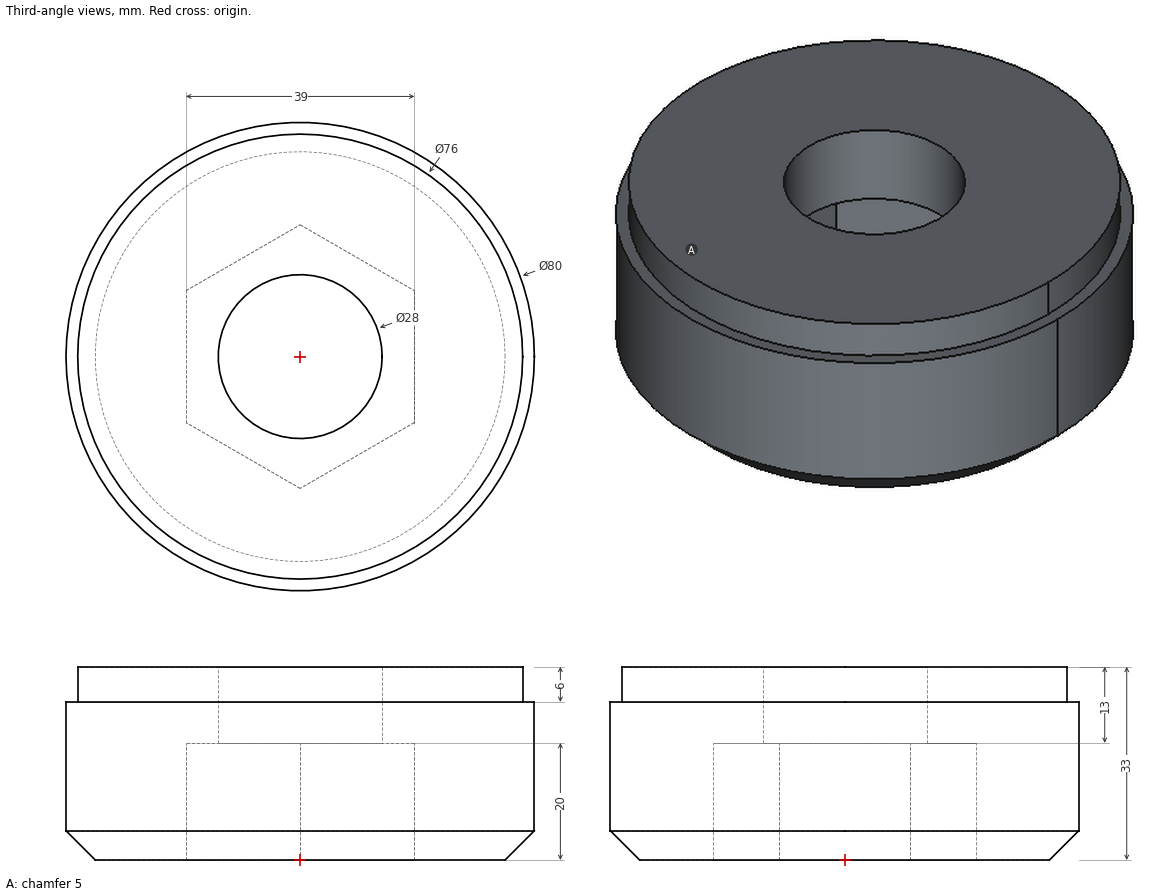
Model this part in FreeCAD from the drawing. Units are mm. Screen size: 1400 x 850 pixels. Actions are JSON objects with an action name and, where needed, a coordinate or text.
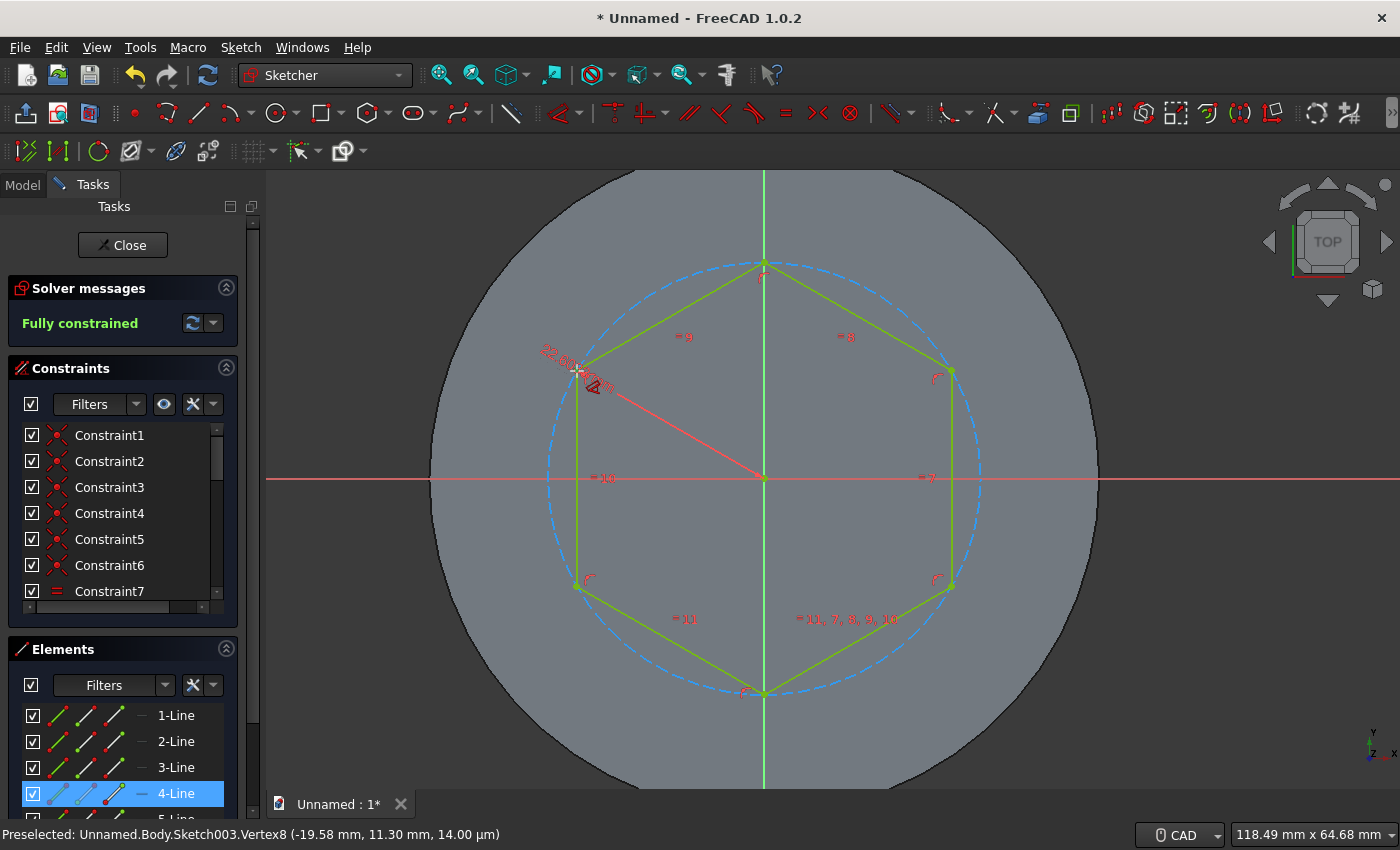
{"action": "left_click", "coordinate": [952, 587]}
{"action": "left_click", "coordinate": [678, 337]}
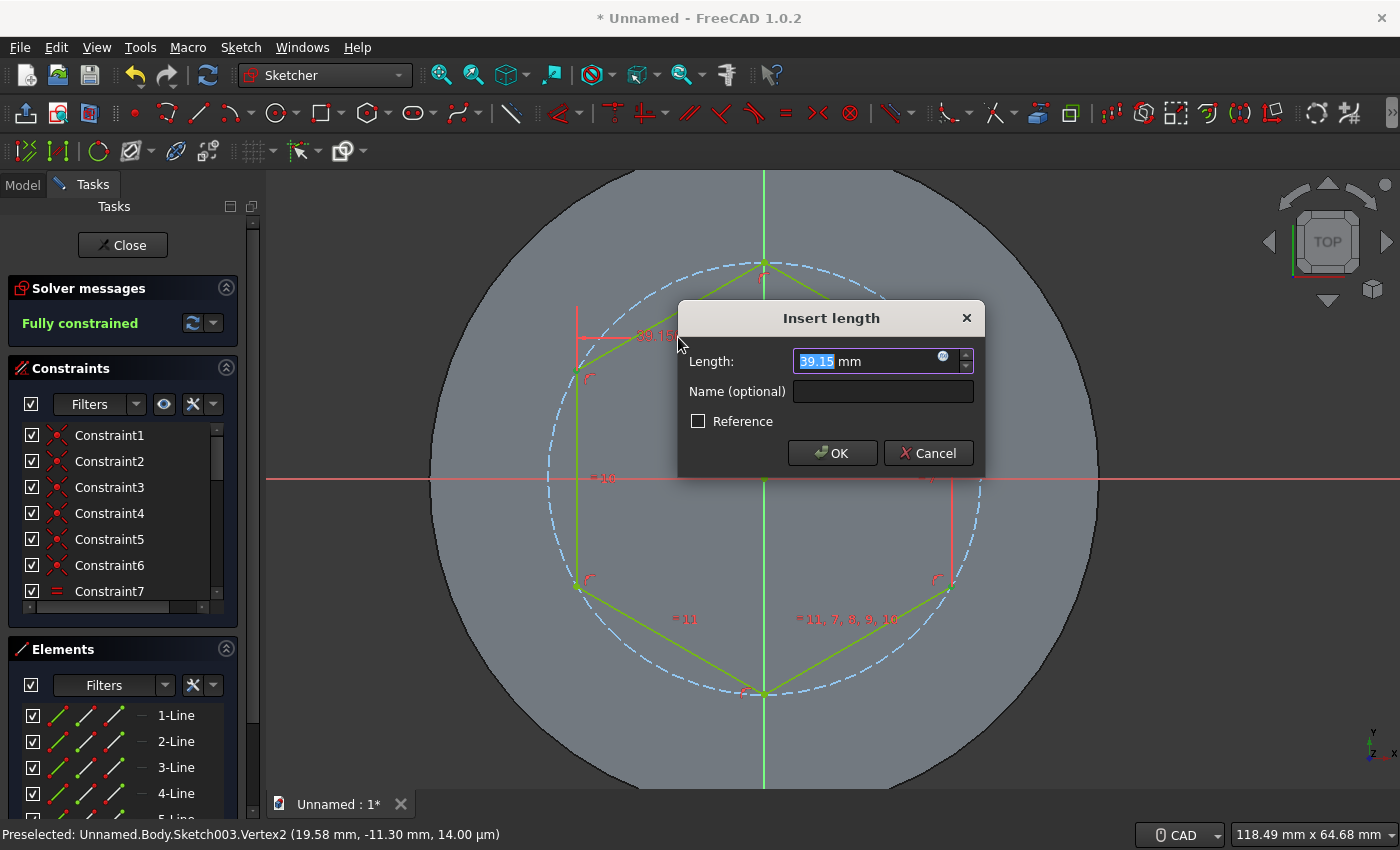
{"action": "type", "text": "39"}
{"action": "key", "text": "Return"}
{"action": "key", "text": "Escape"}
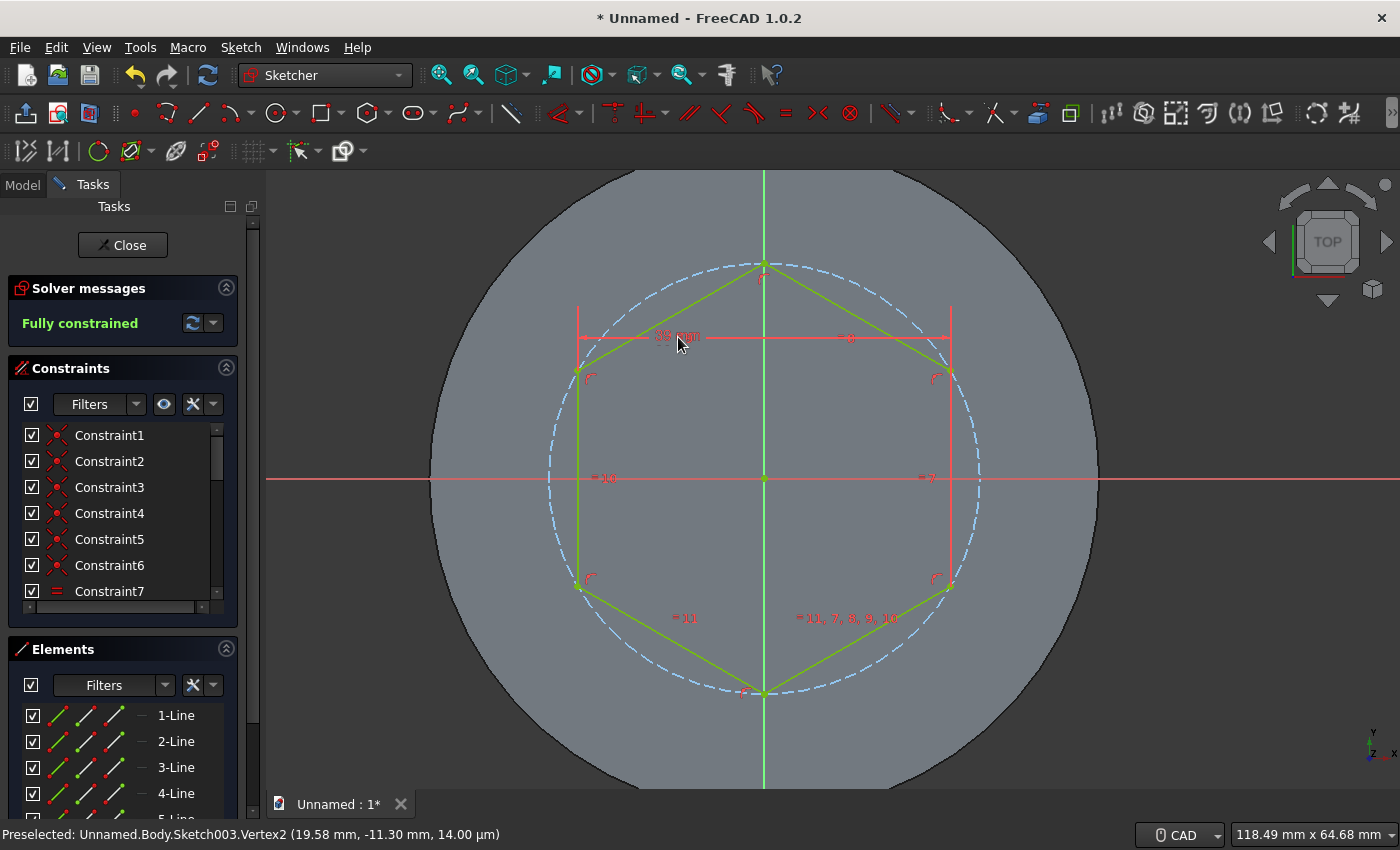
{"action": "left_click", "coordinate": [123, 245]}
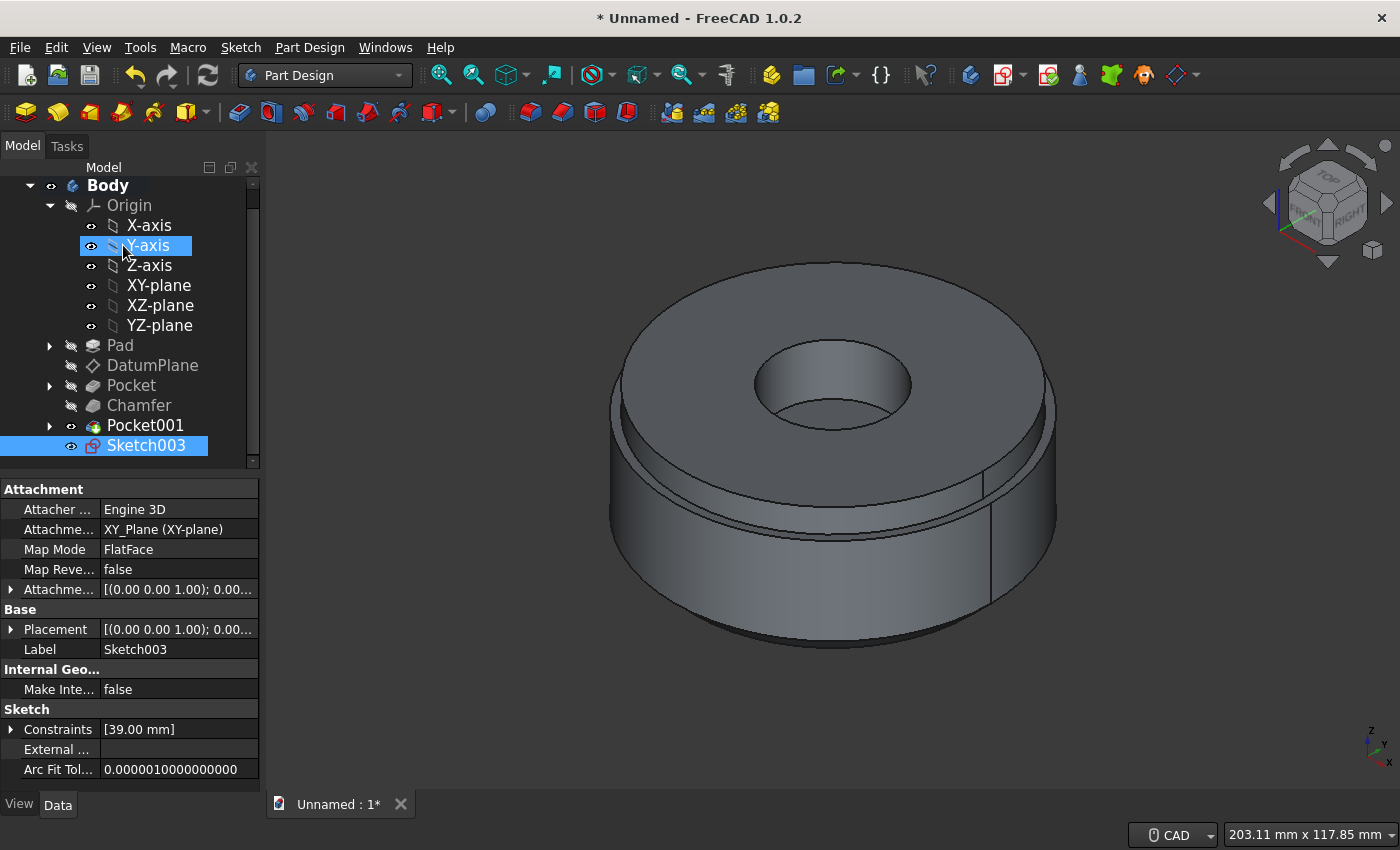
{"action": "left_click", "coordinate": [240, 112]}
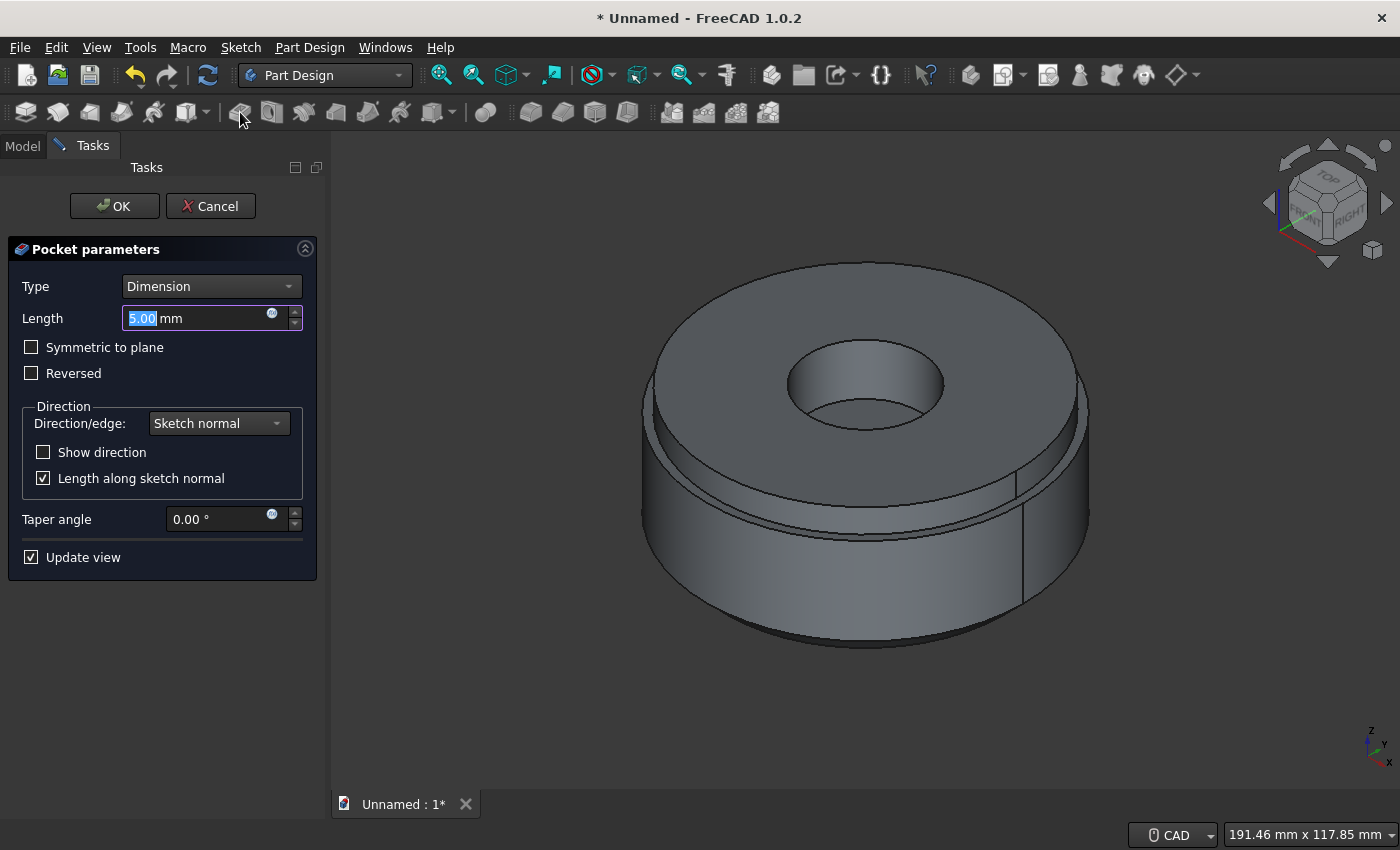
{"action": "type", "text": "20"}
{"action": "key", "text": "Tab"}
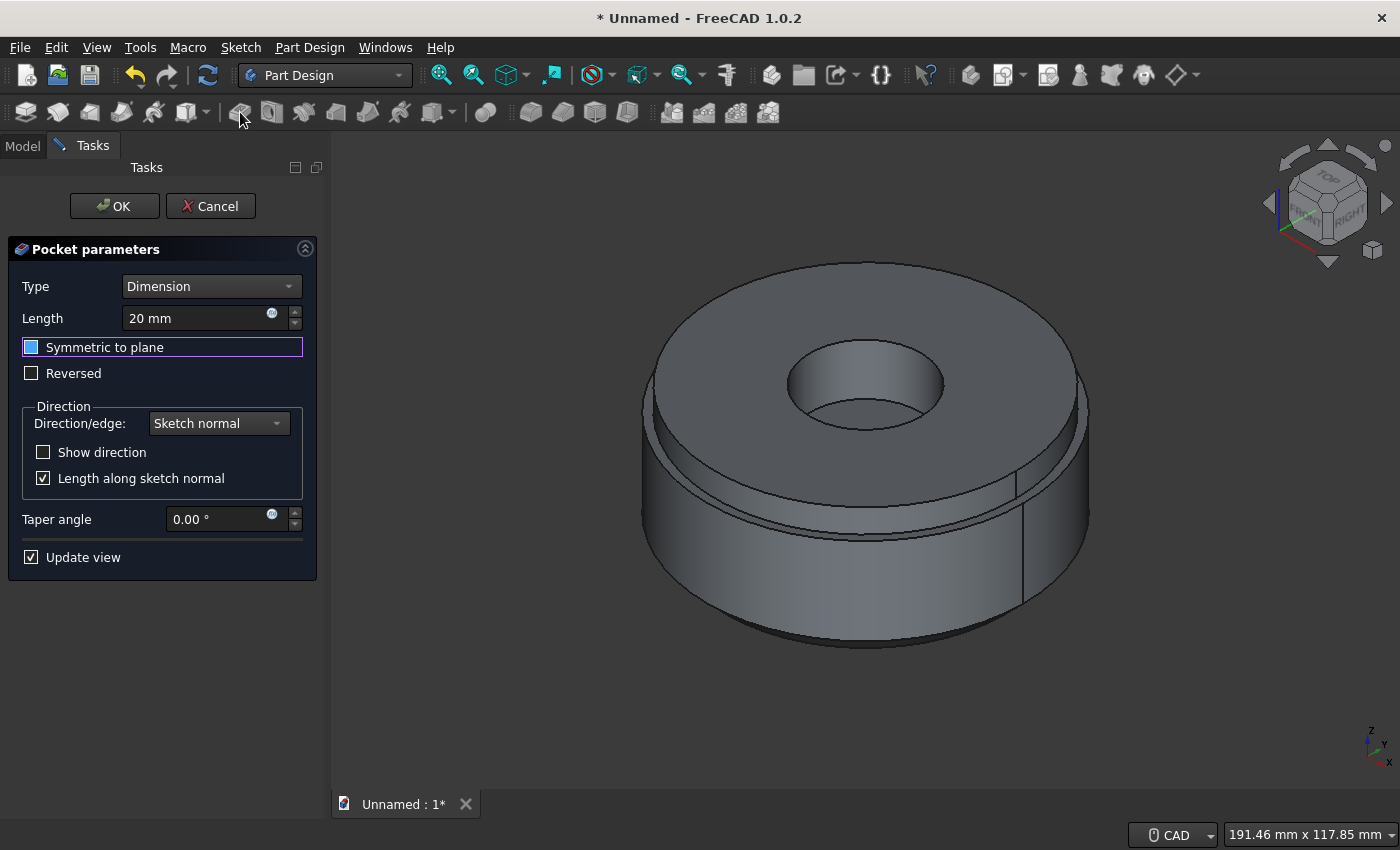
{"action": "left_click", "coordinate": [30, 373]}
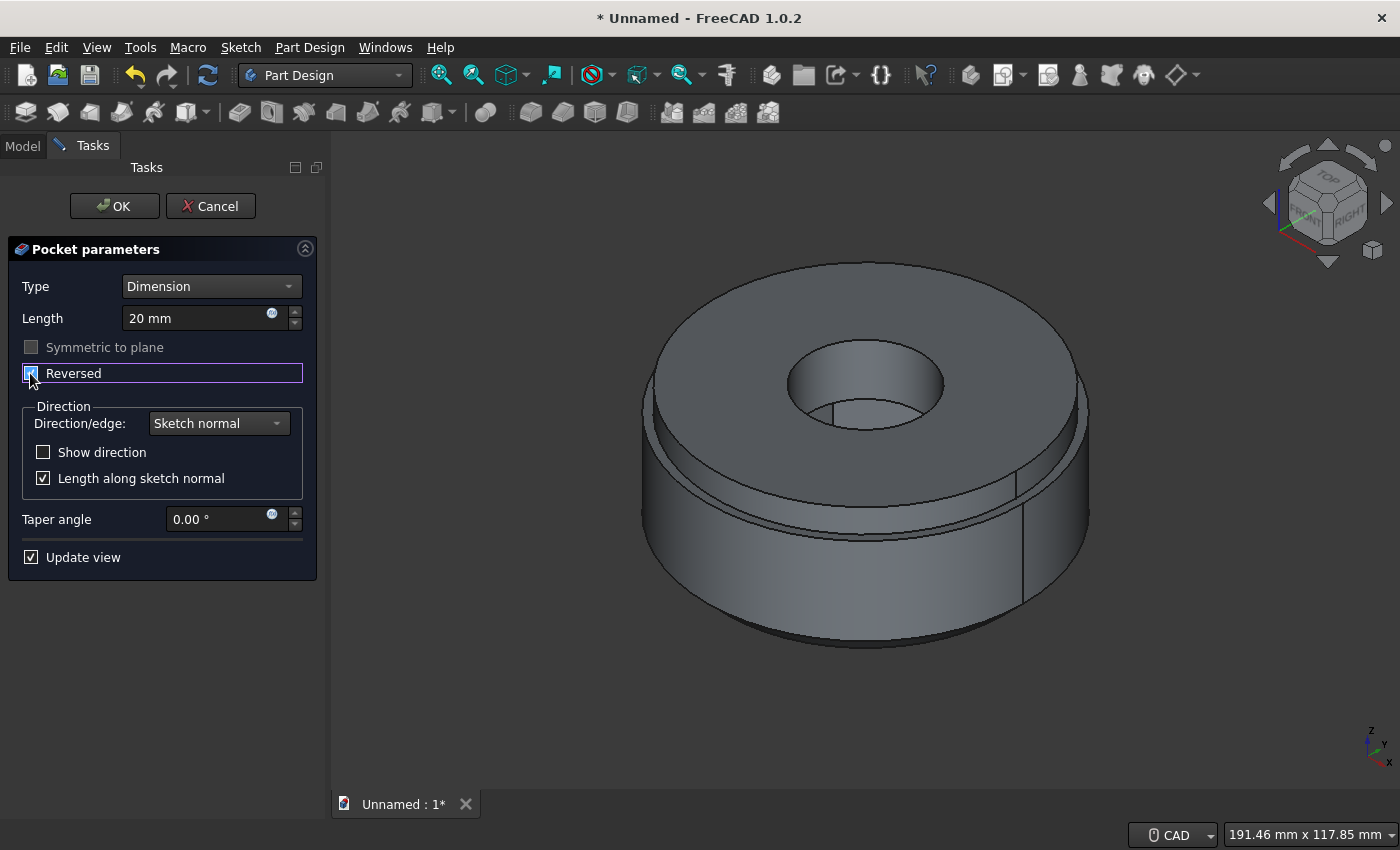
{"action": "left_click", "coordinate": [115, 206]}